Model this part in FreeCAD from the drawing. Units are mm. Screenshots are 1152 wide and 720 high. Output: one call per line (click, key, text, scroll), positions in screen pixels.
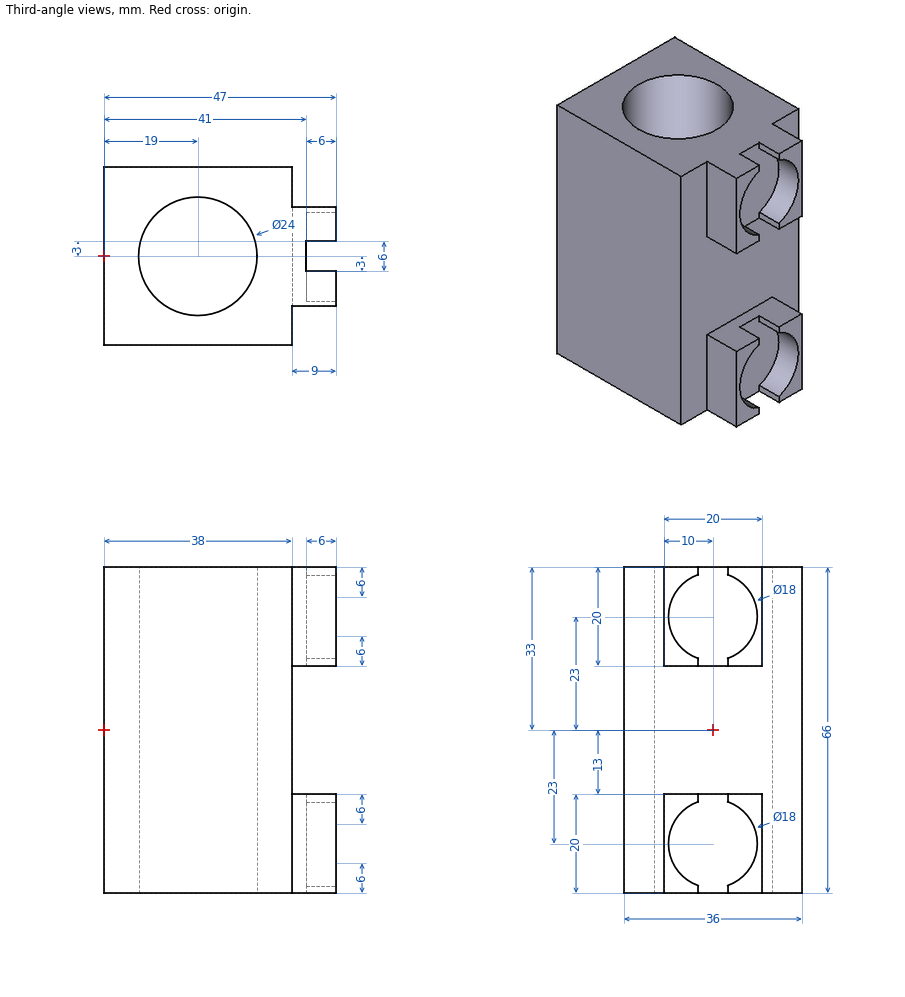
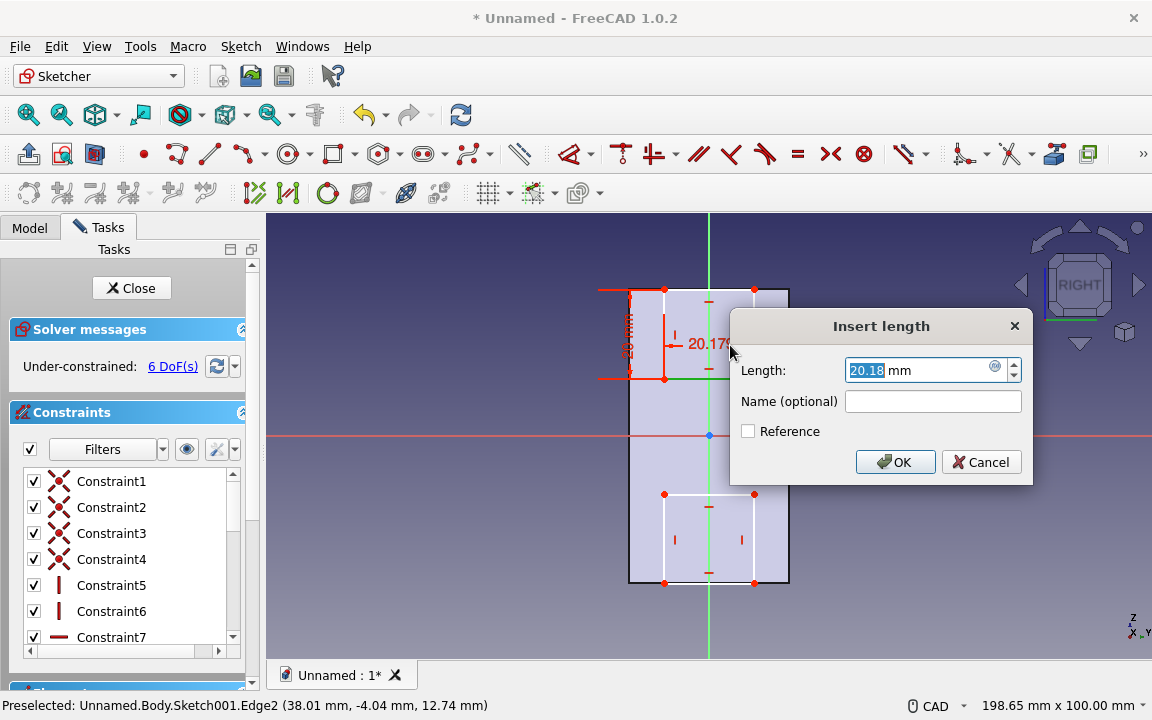
text(20)
key(Return)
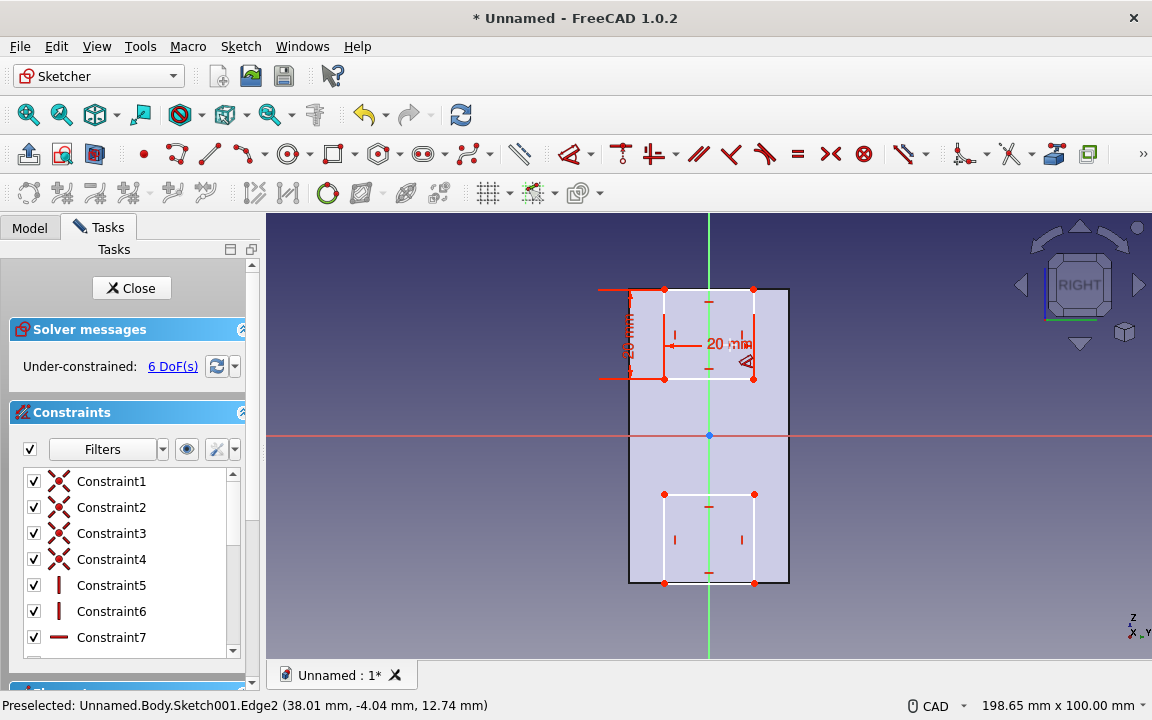
click(664, 522)
click(630, 540)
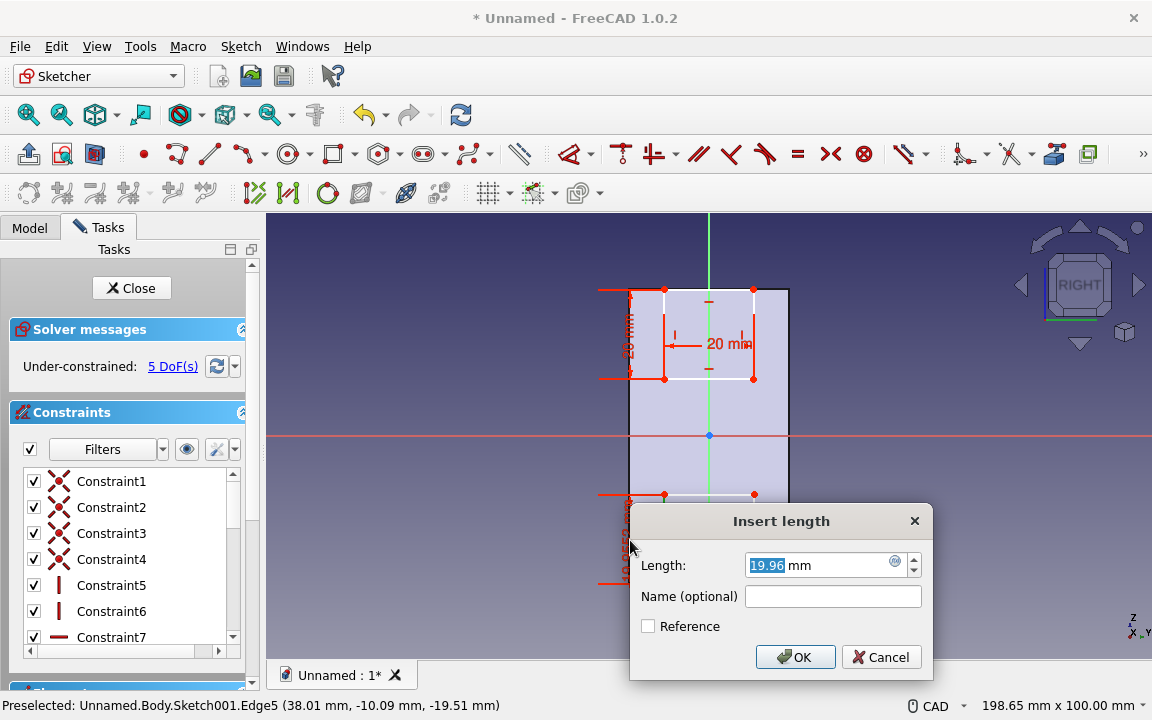
text(20)
key(Return)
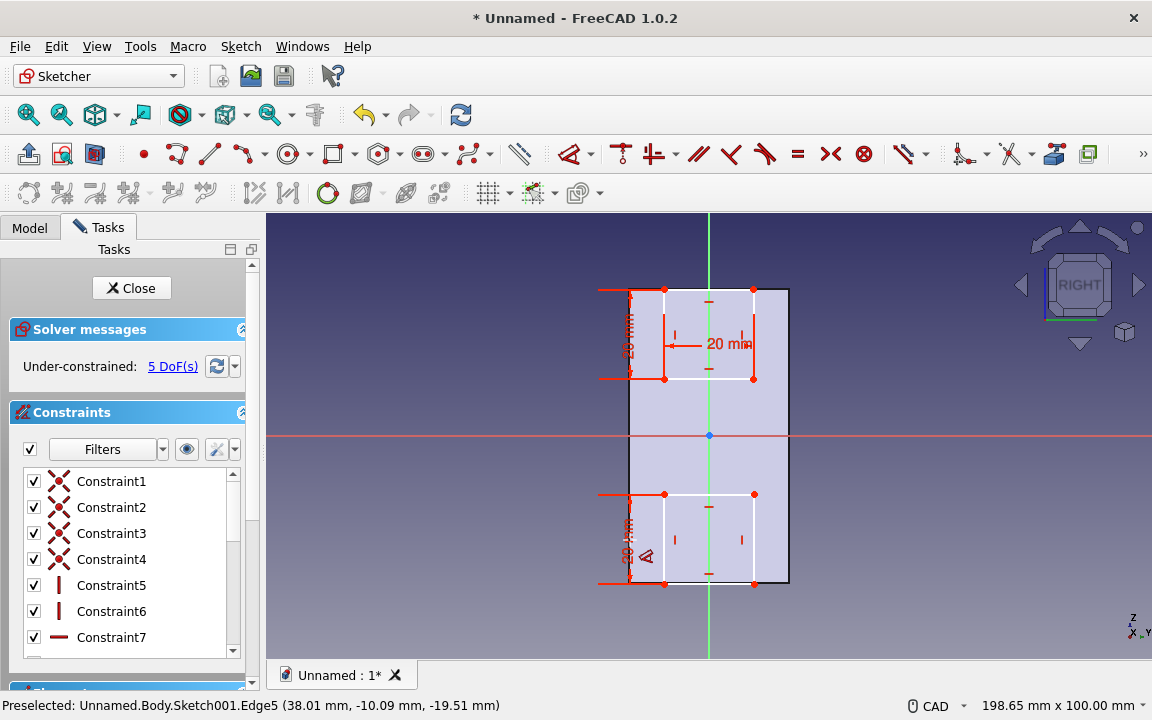
click(691, 584)
click(688, 618)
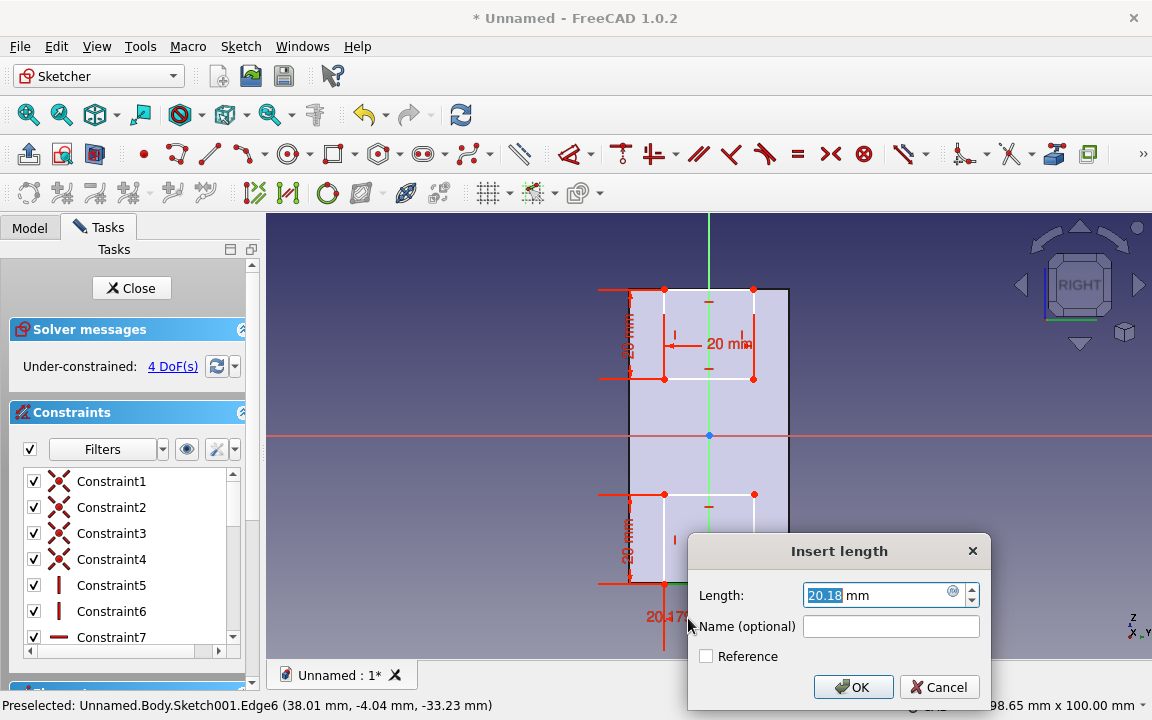
text(20)
key(Return)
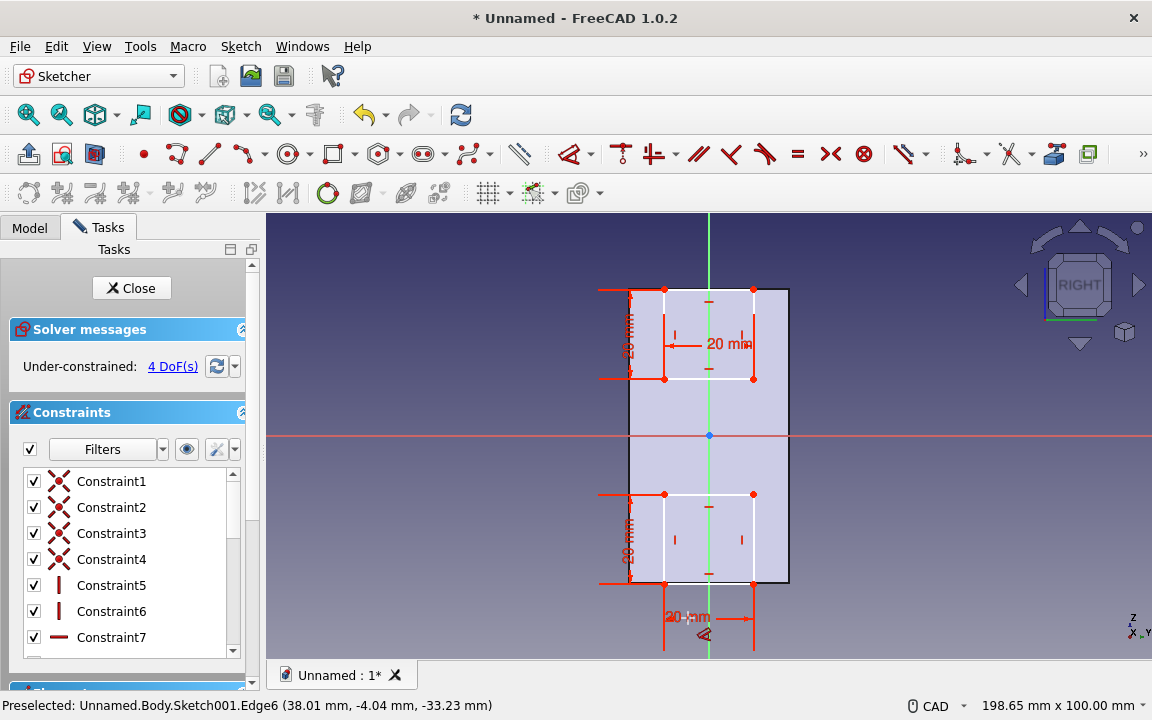
click(664, 290)
click(687, 256)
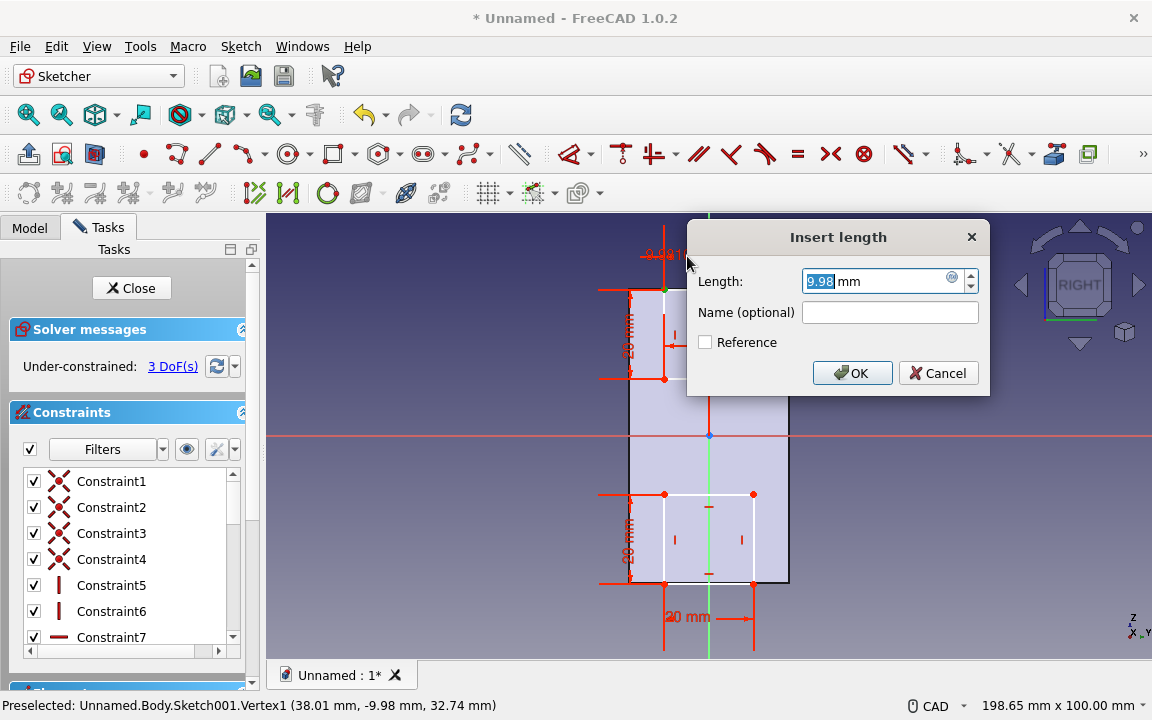
text(10)
key(Return)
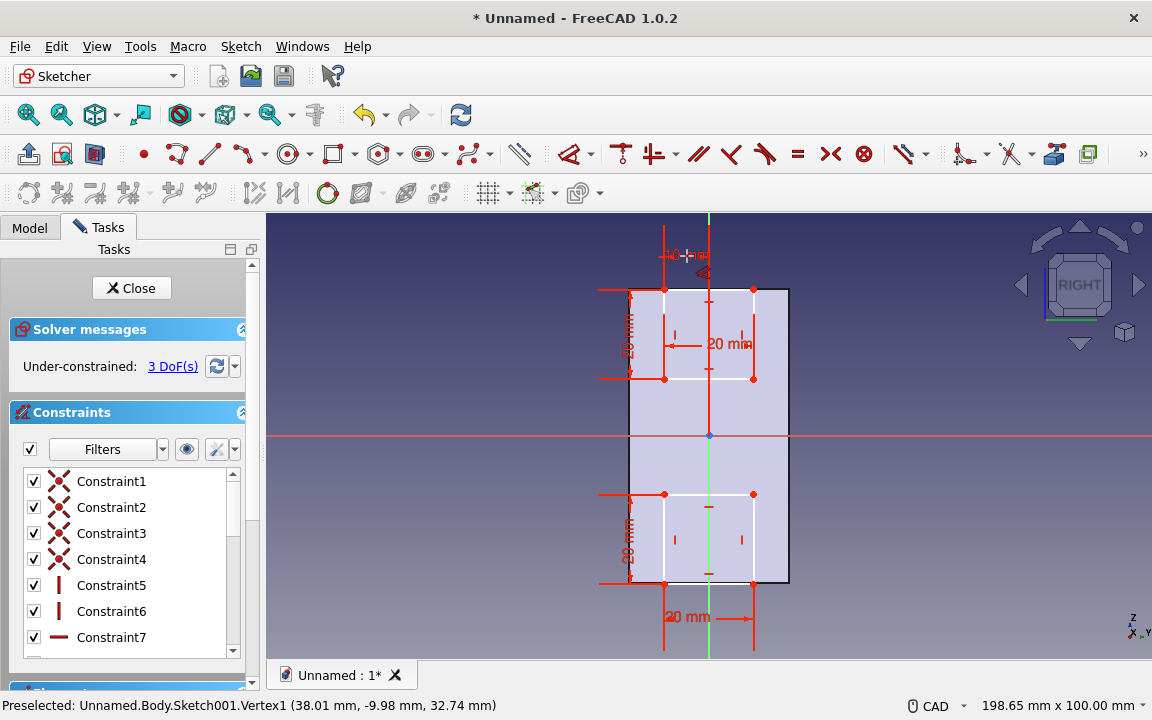
click(664, 290)
click(630, 363)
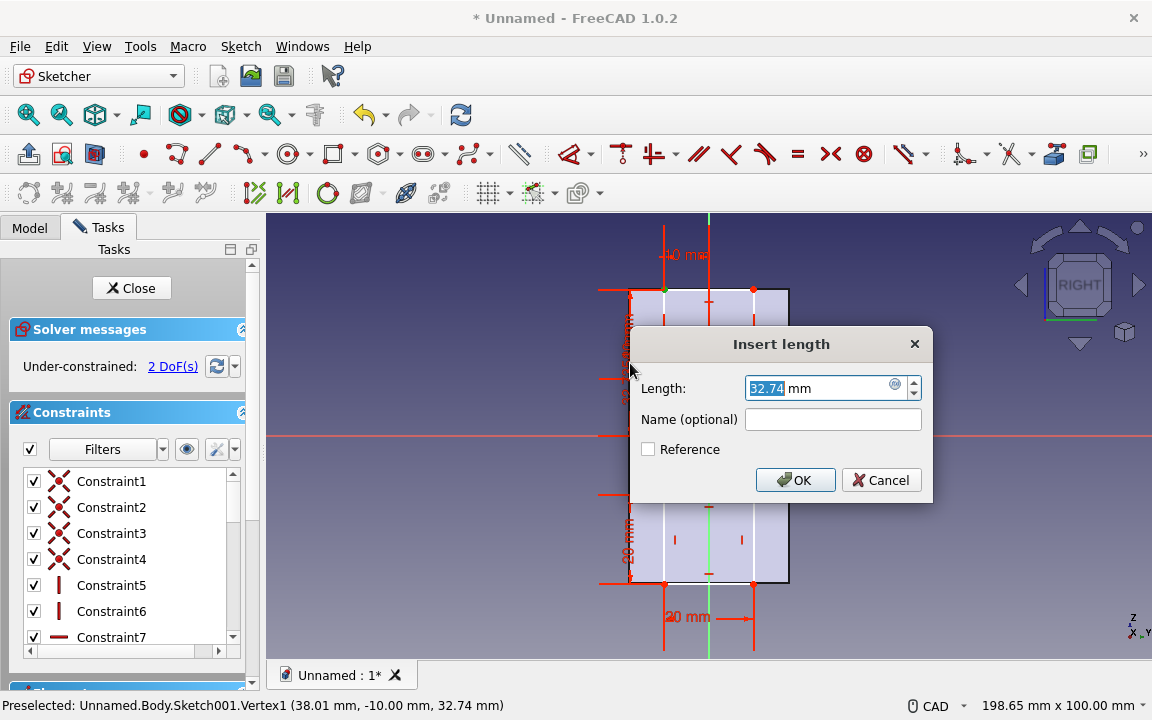
text(33)
key(Return)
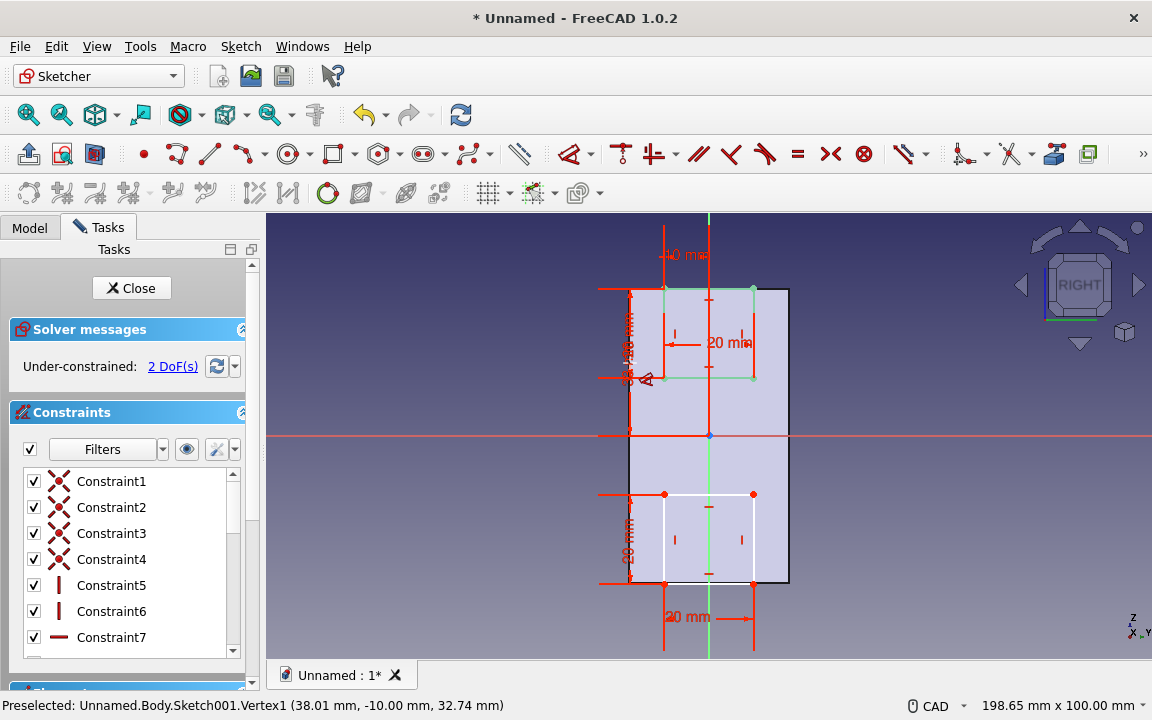
click(664, 495)
click(687, 402)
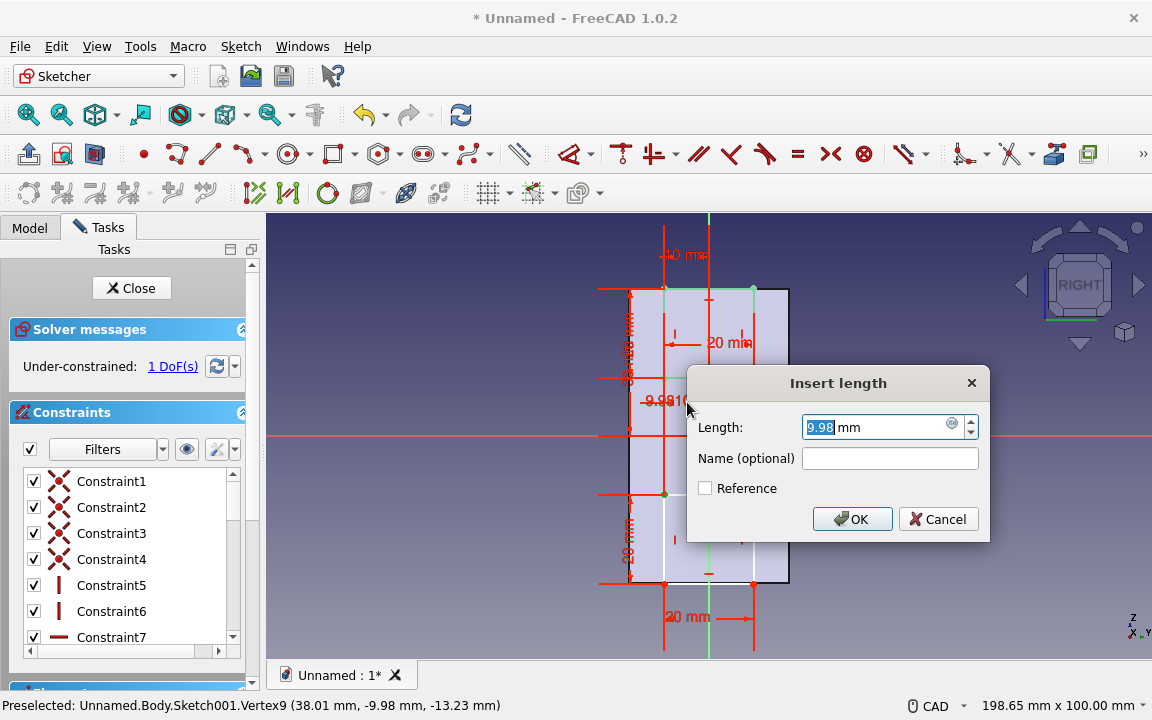
text(10)
key(Return)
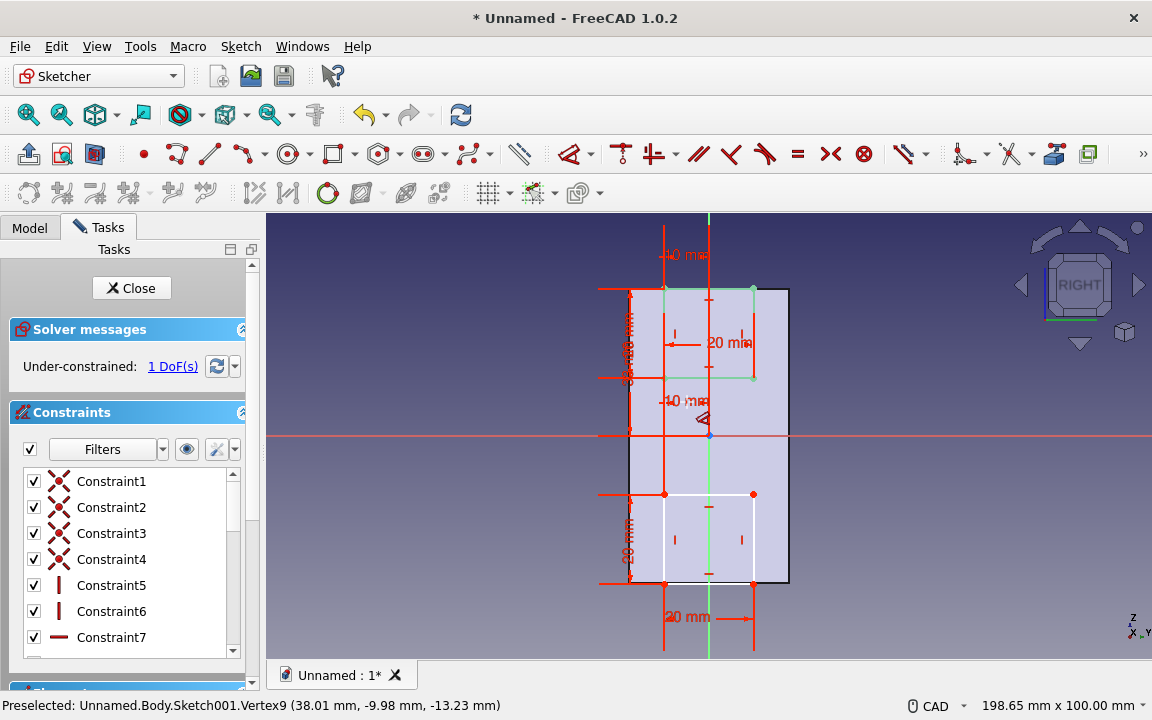
click(664, 495)
click(630, 466)